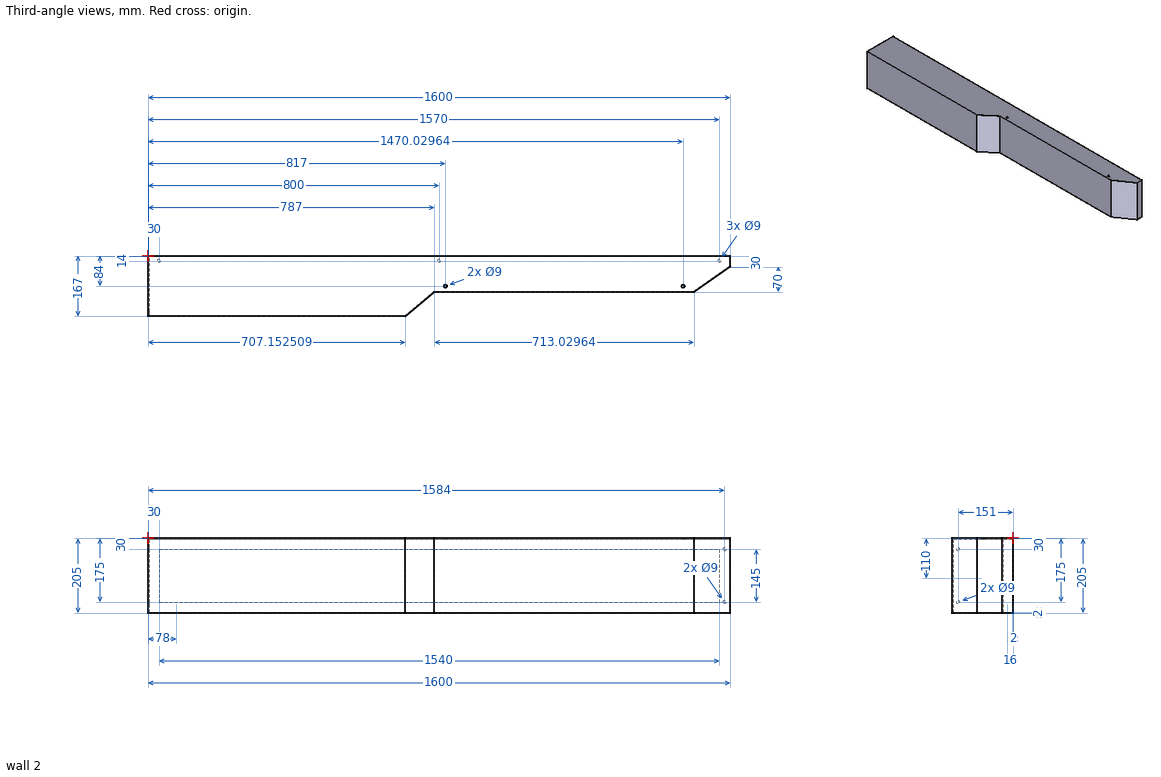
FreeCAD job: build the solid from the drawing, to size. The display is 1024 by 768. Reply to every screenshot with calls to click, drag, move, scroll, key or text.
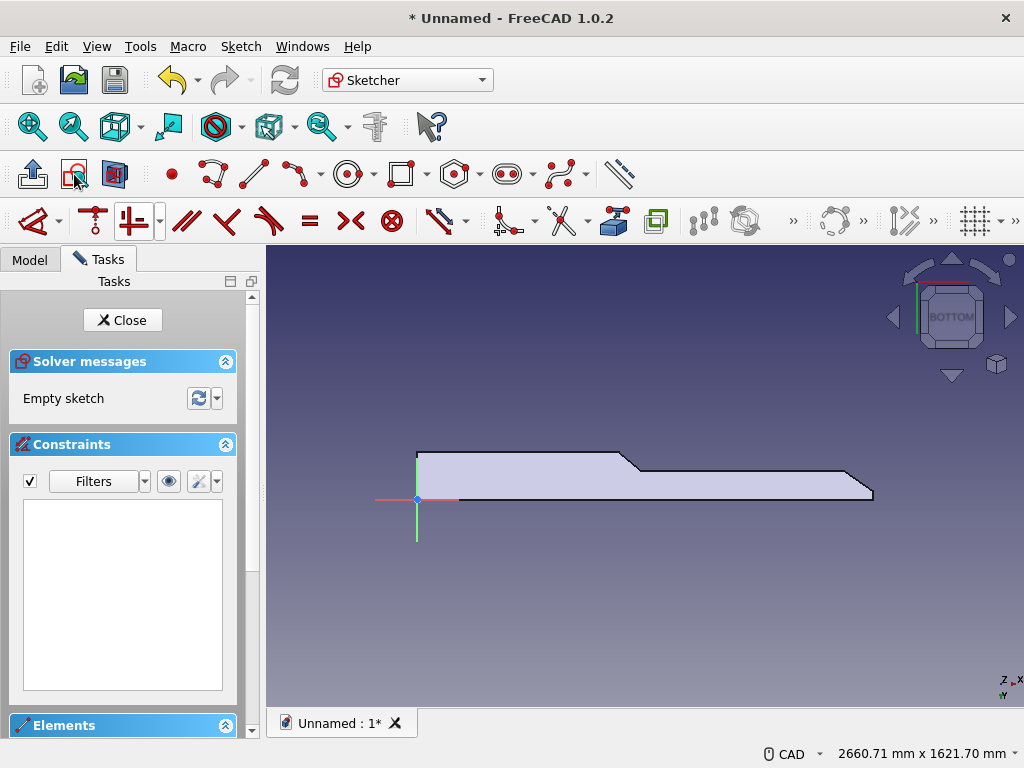
scroll(294, 380, down, 1)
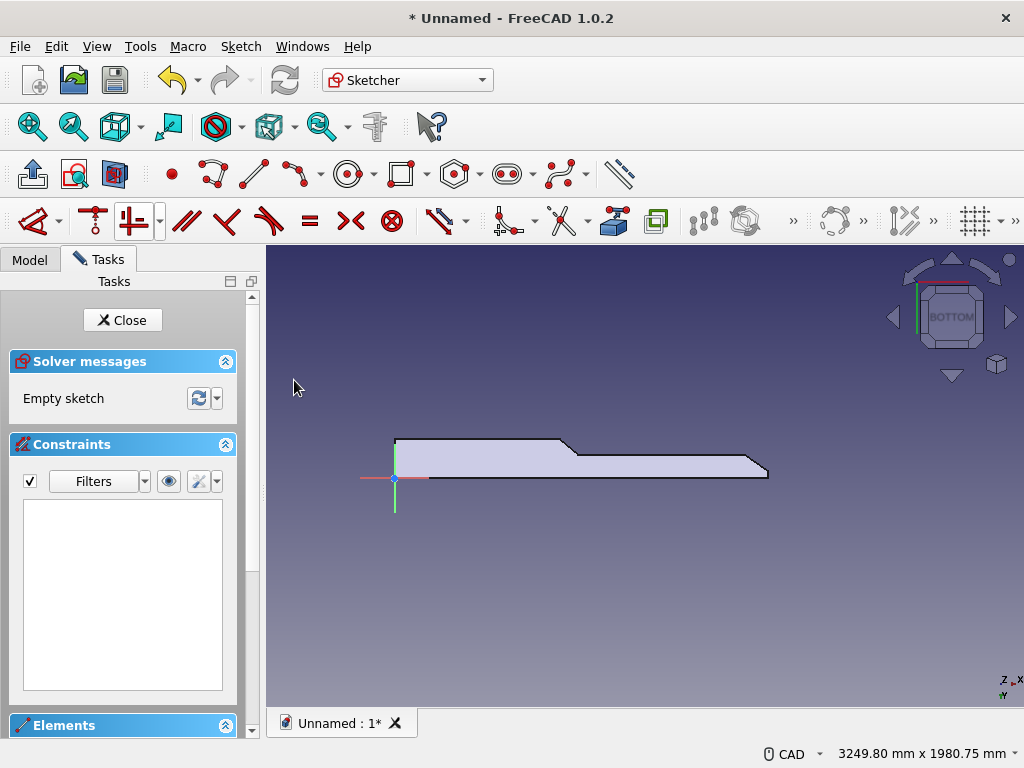
key(g)
key(c)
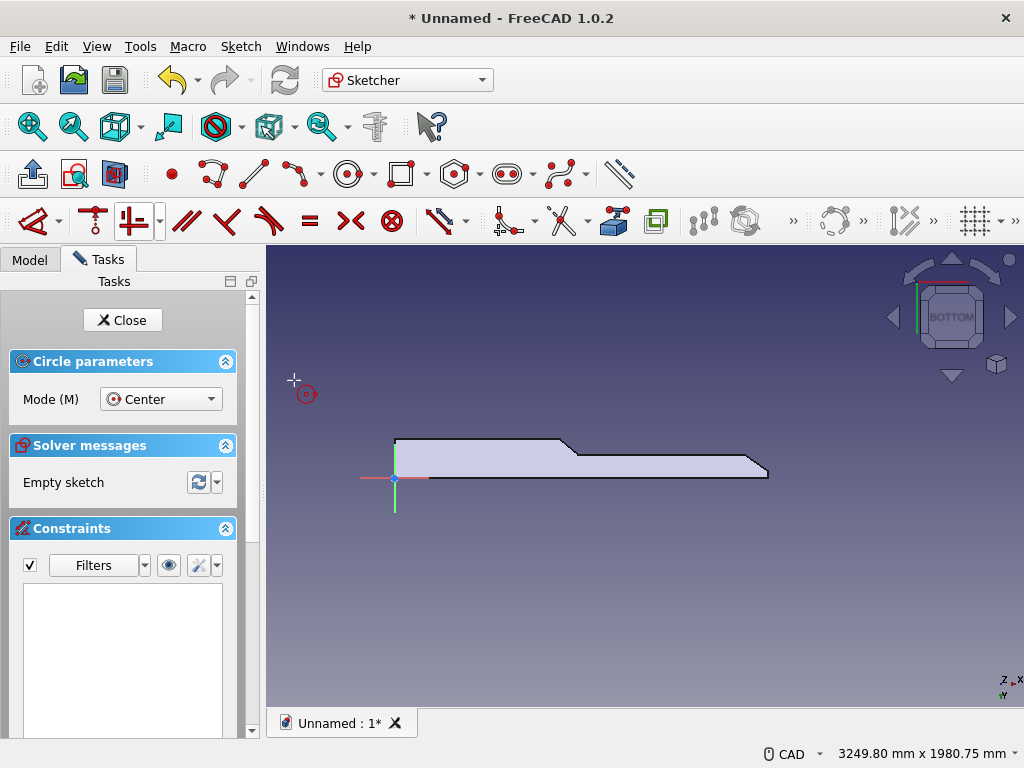
scroll(761, 475, up, 16)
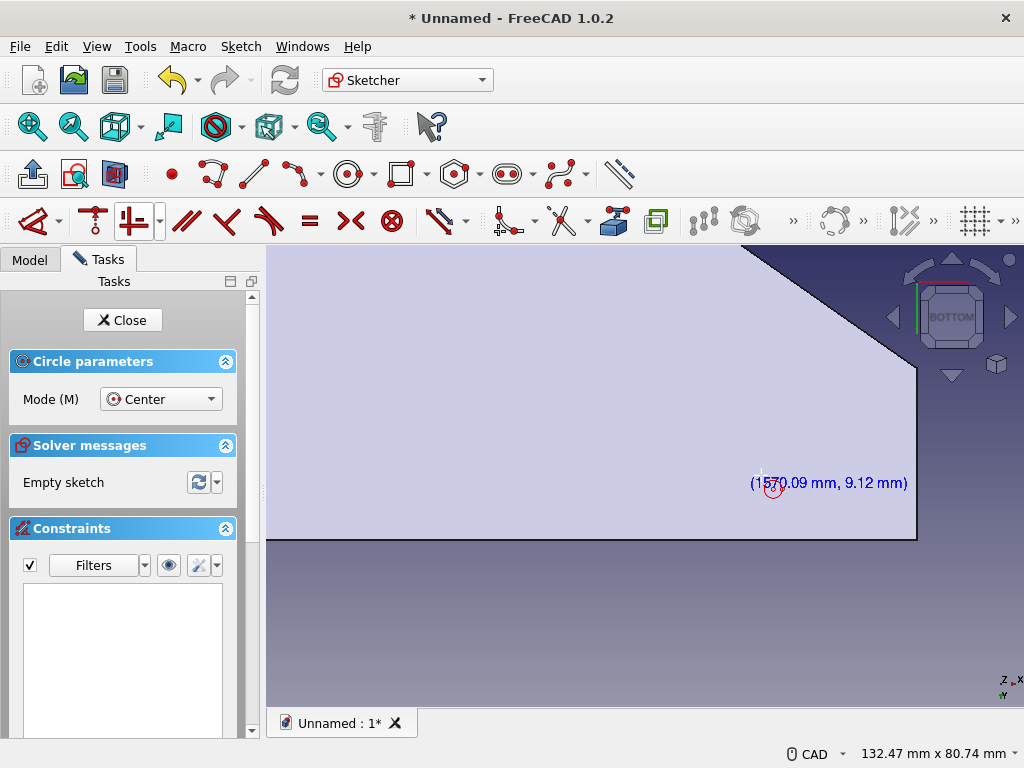
scroll(802, 475, down, 15)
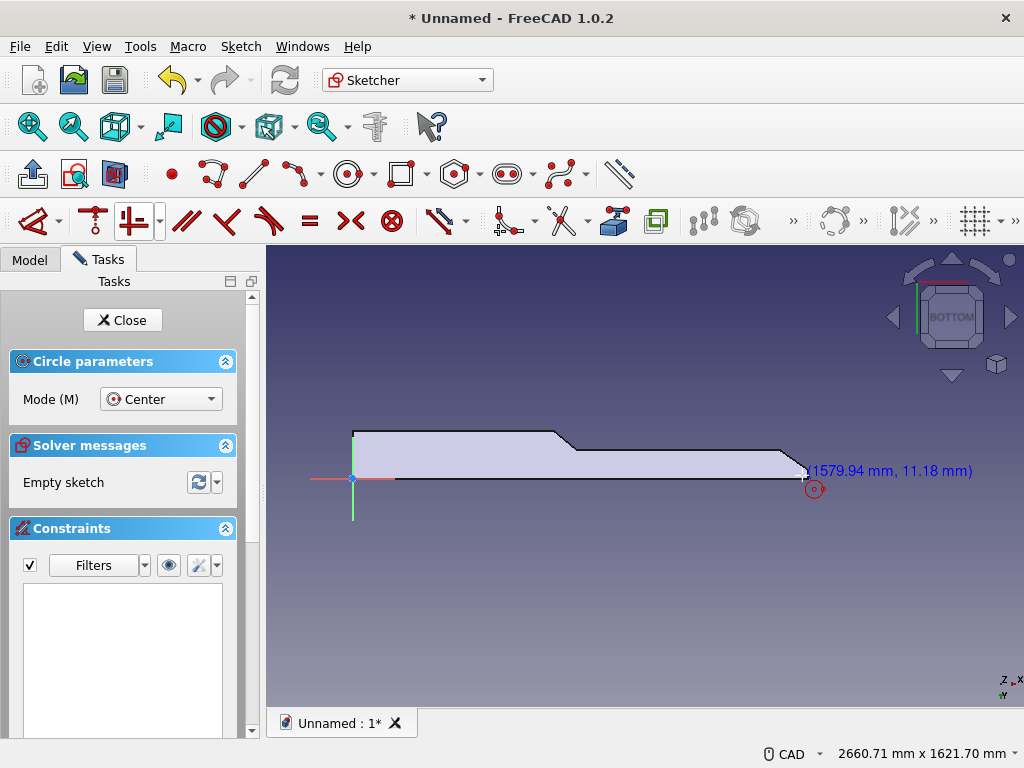
scroll(800, 475, up, 7)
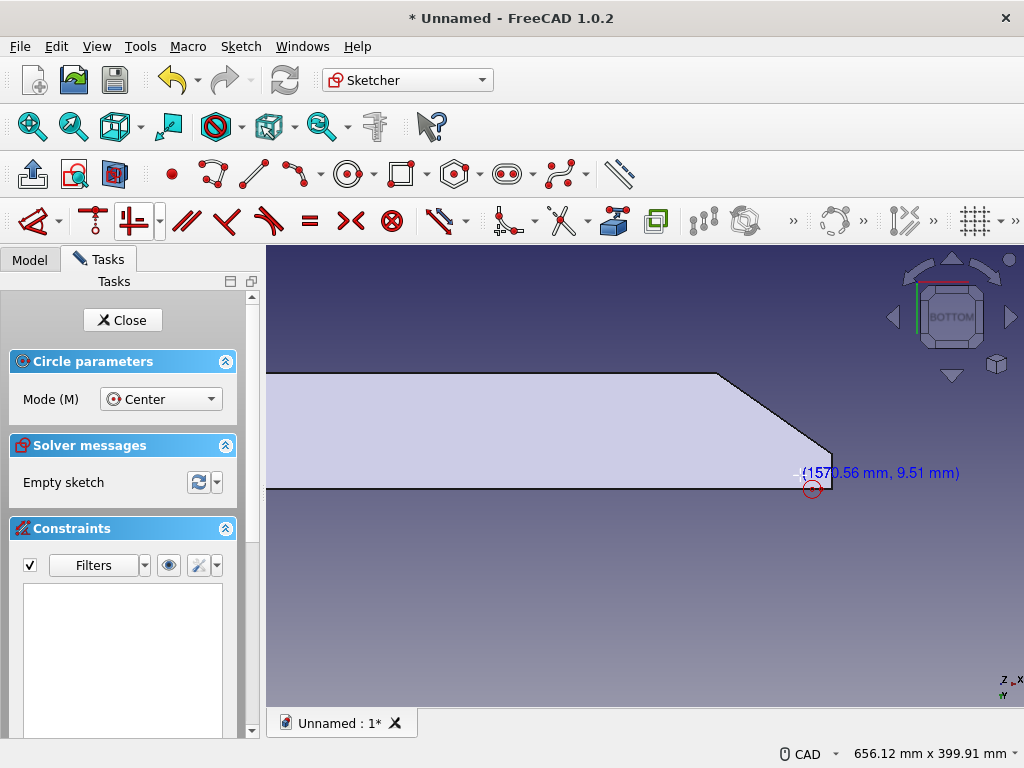
click(797, 472)
move(801, 469)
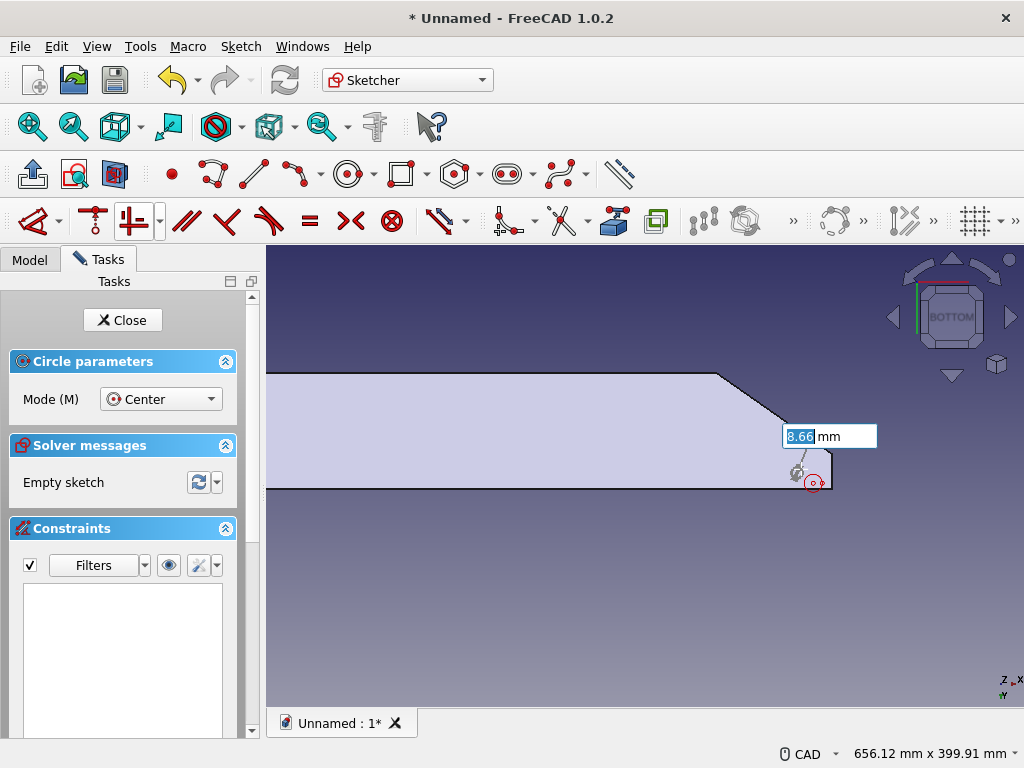
text(9)
key(Return)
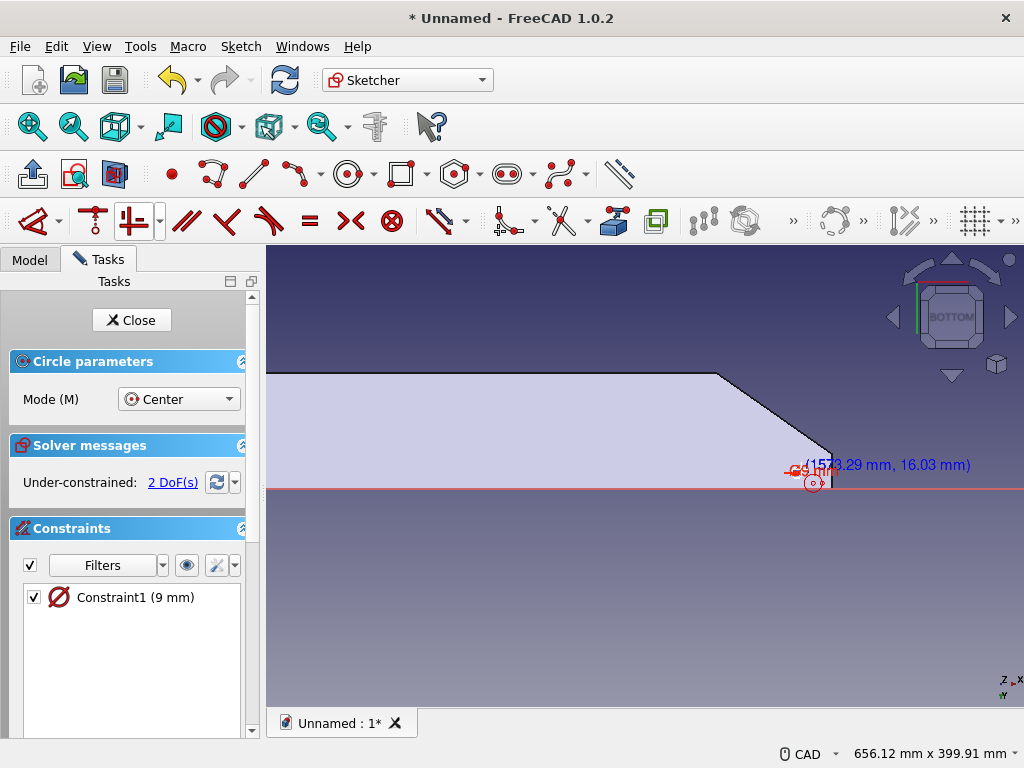
scroll(749, 476, down, 8)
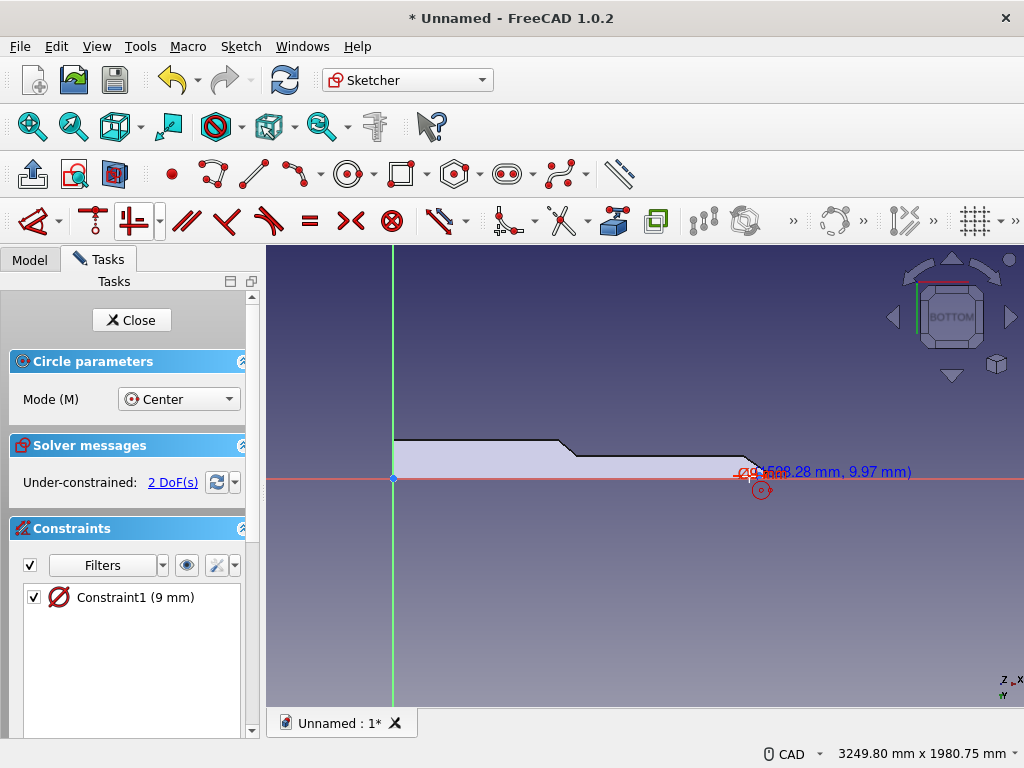
scroll(400, 476, up, 16)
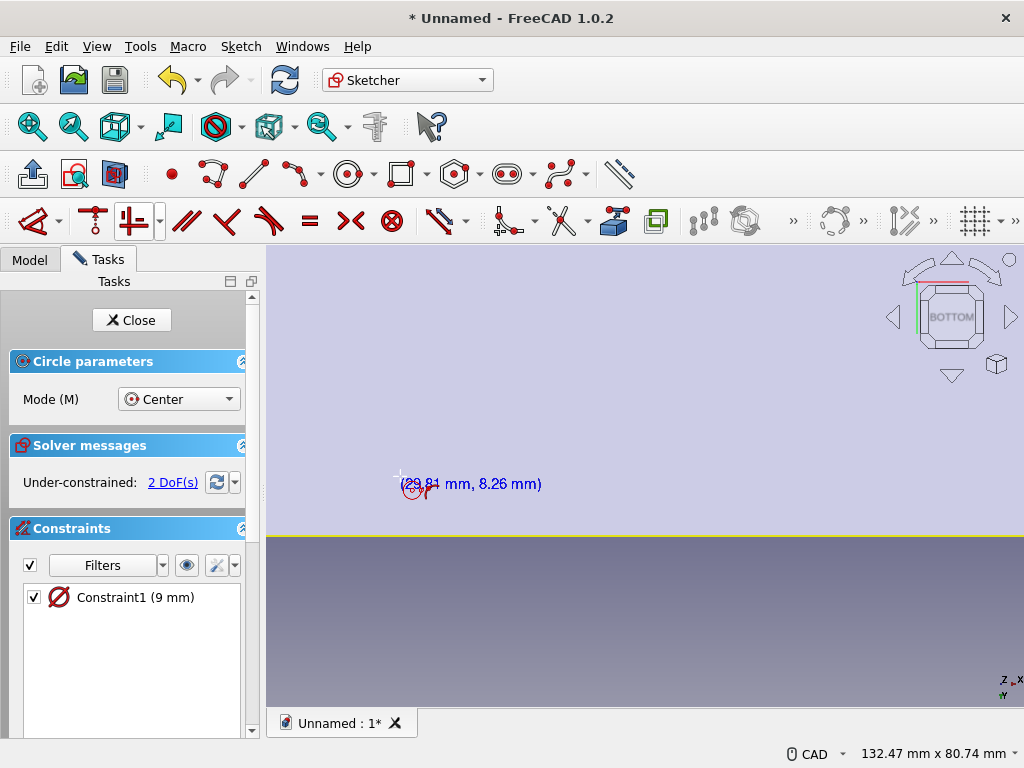
scroll(359, 476, down, 15)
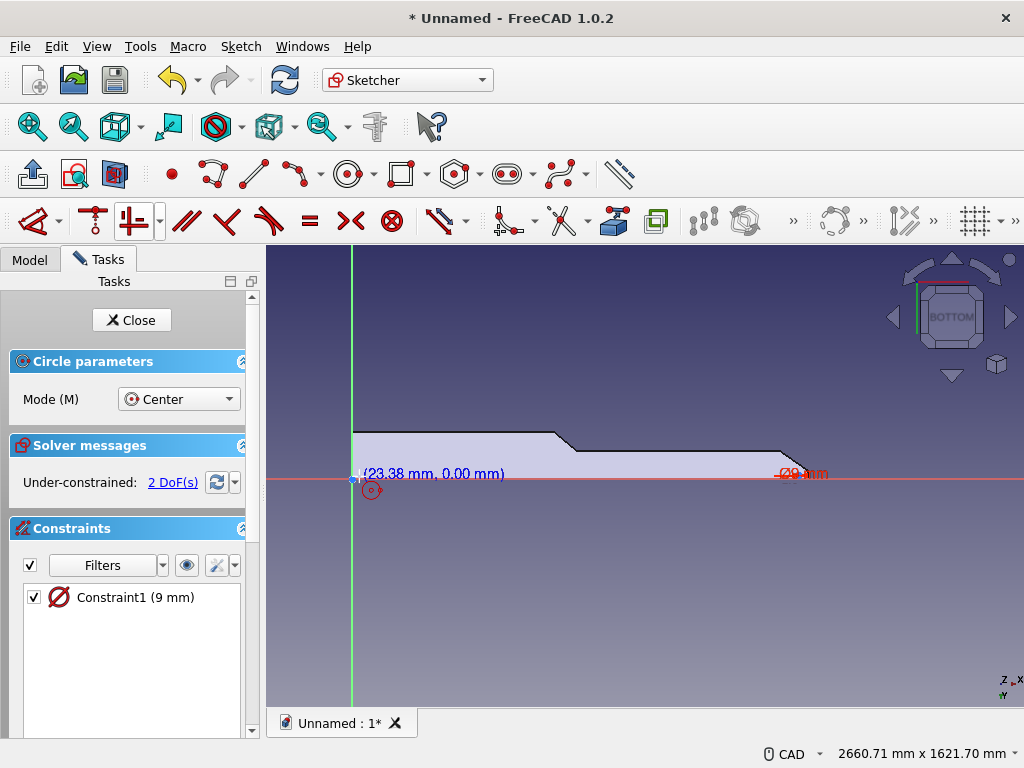
scroll(361, 475, up, 7)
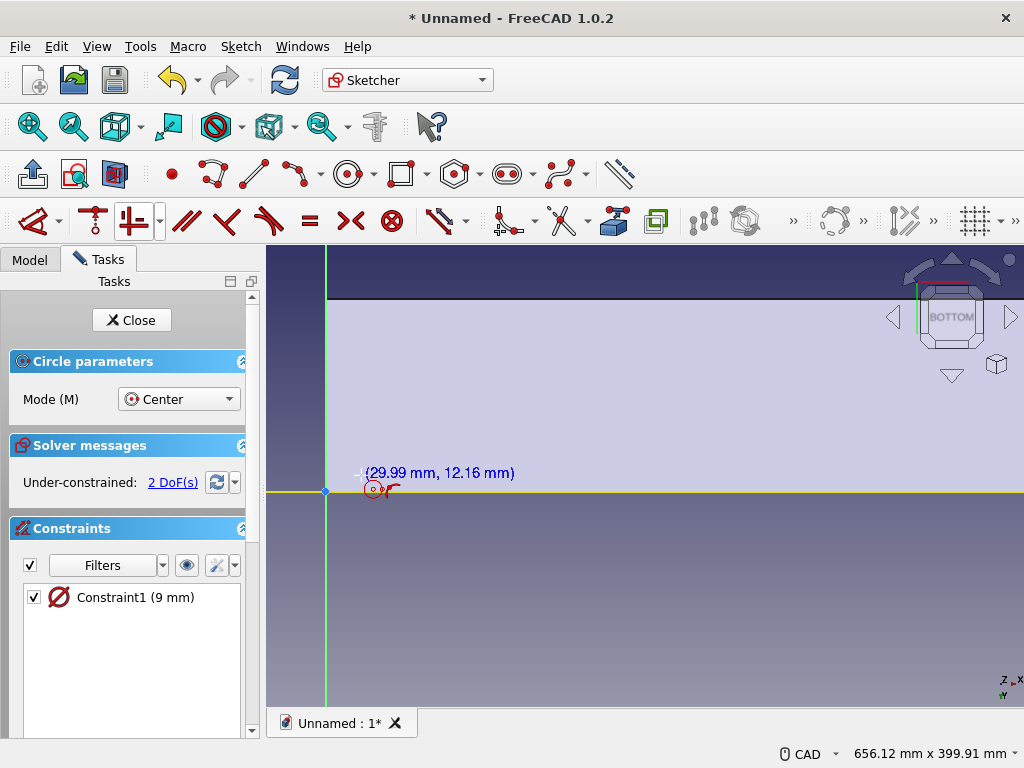
click(361, 475)
move(364, 472)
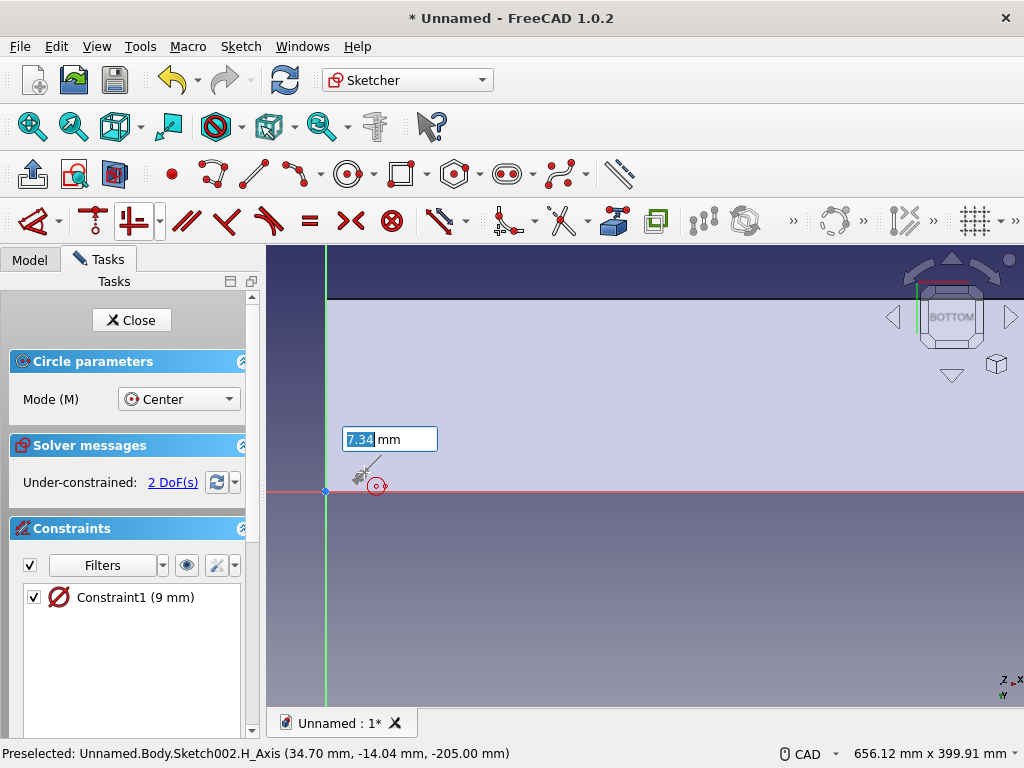
text(9)
key(Return)